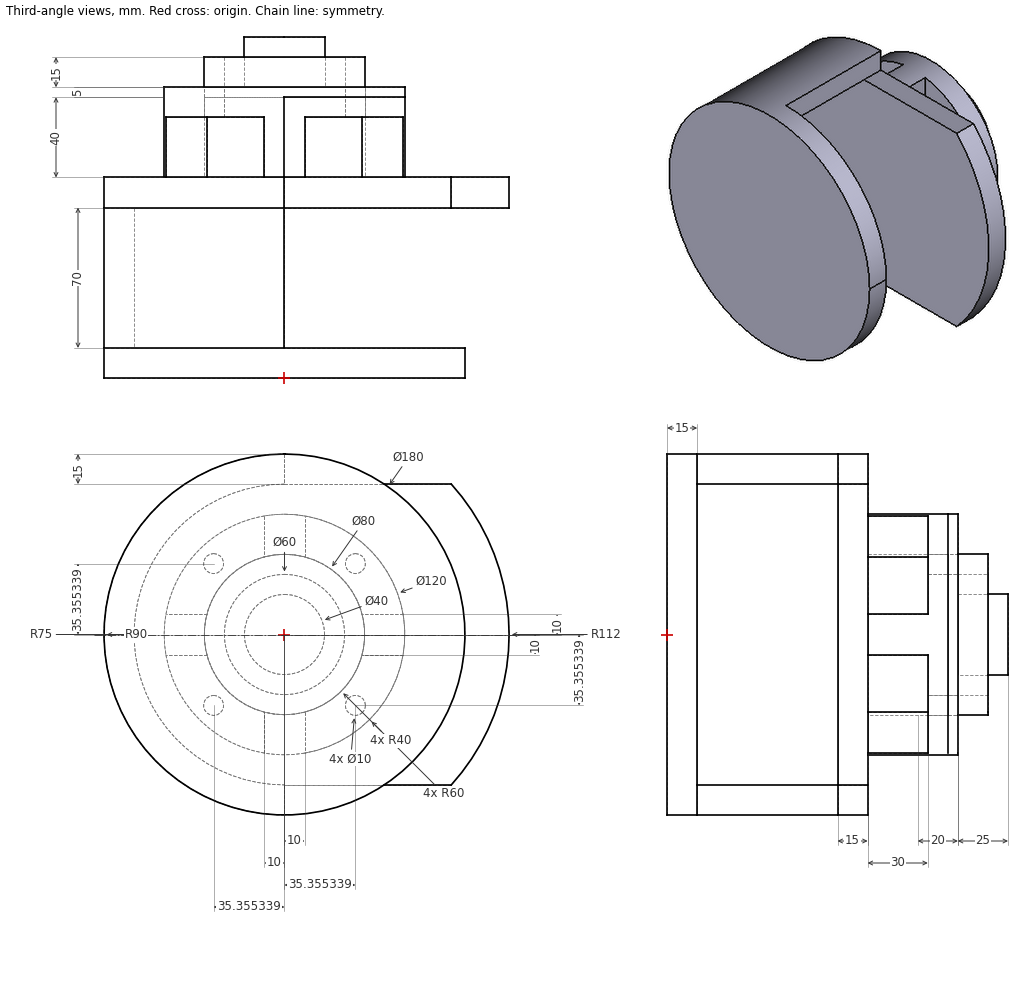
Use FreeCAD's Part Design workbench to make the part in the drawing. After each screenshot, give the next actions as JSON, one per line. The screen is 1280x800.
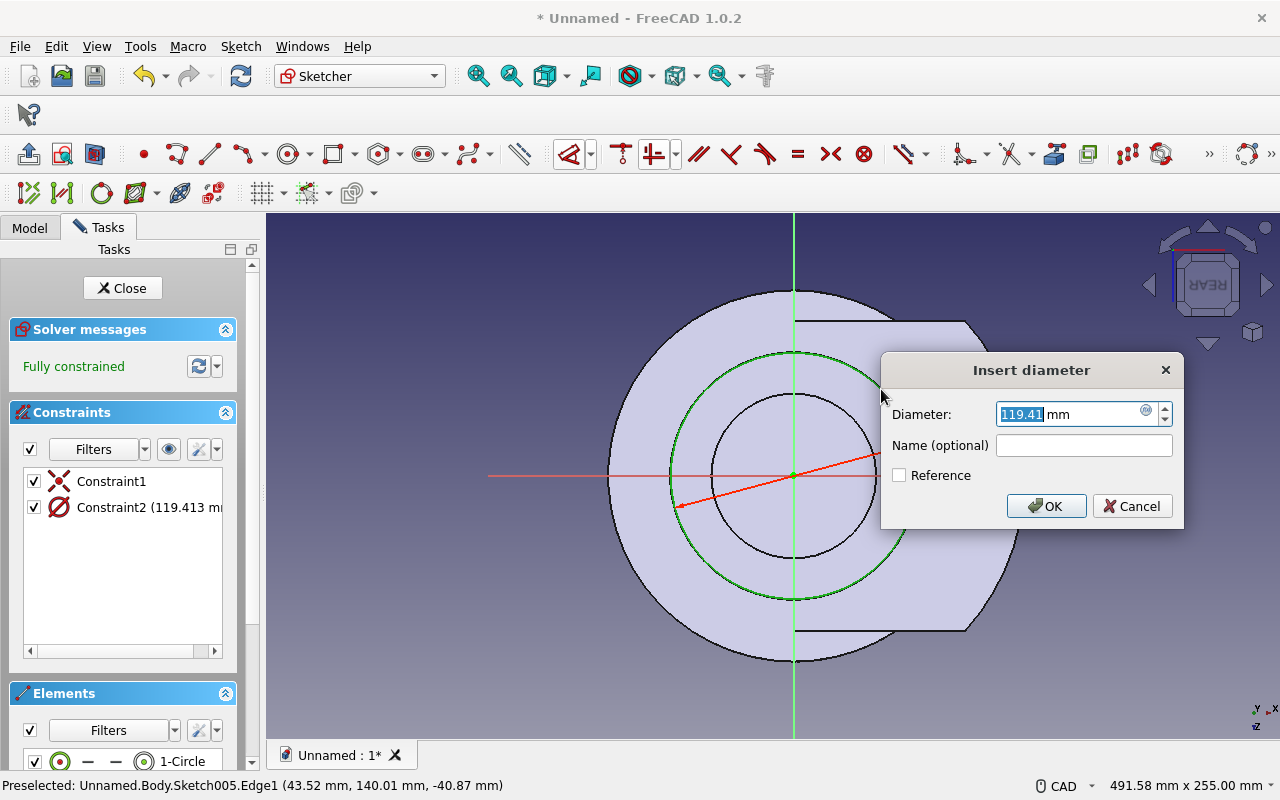
{"action": "type", "text": "120"}
{"action": "key", "text": "Return"}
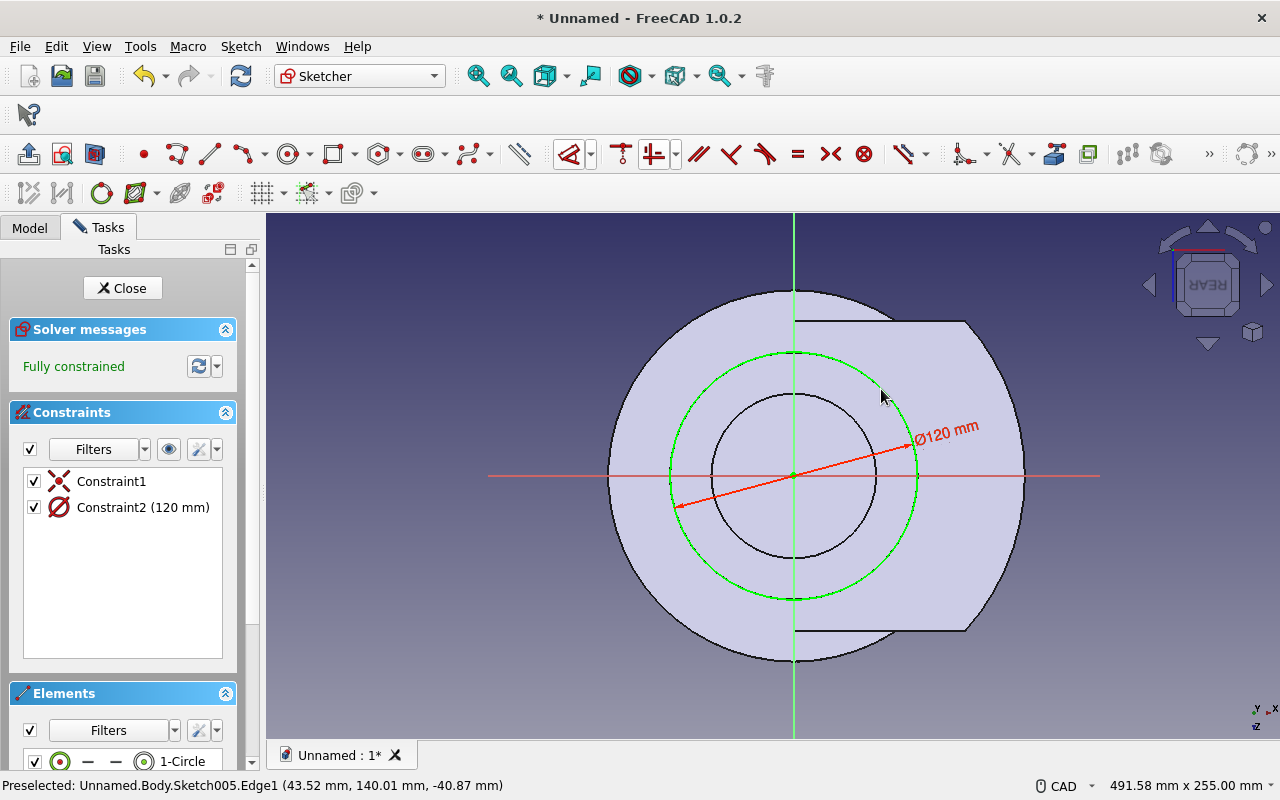
{"action": "left_click", "coordinate": [123, 288]}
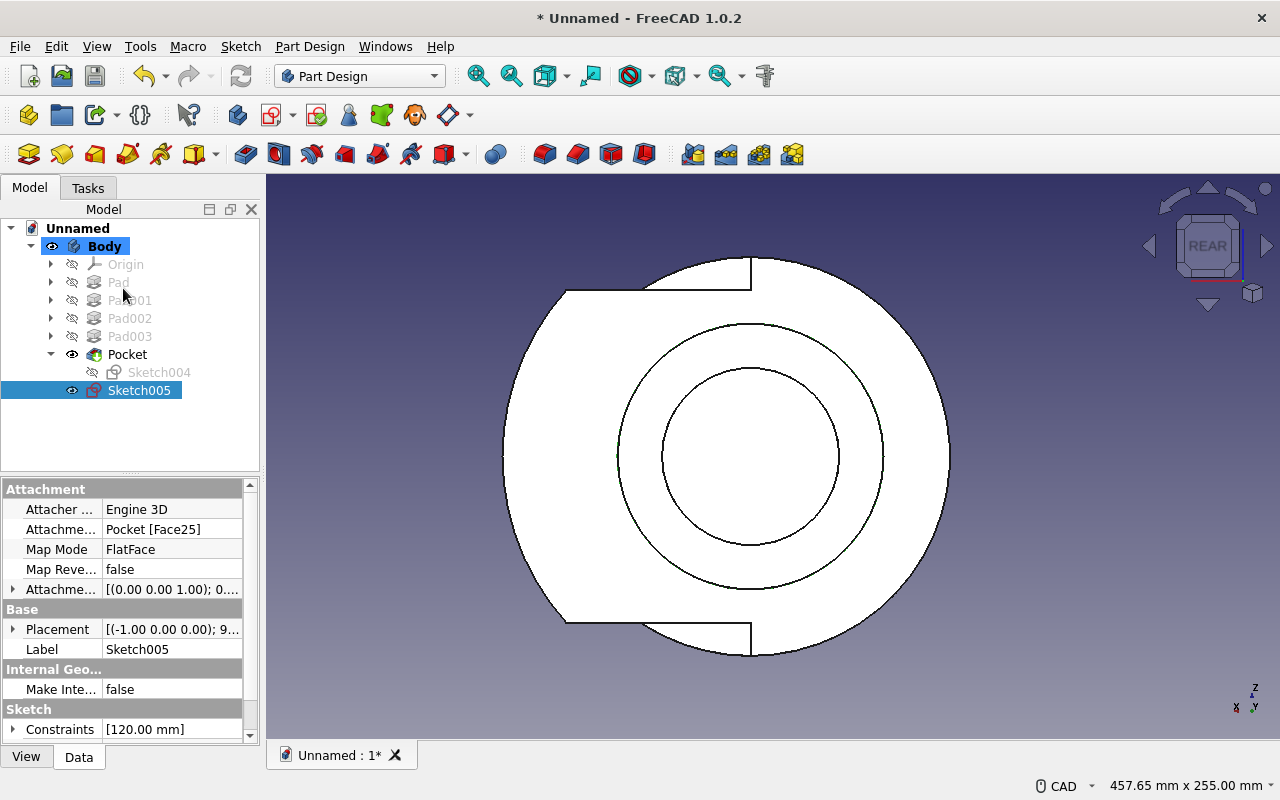
{"action": "left_click", "coordinate": [29, 154]}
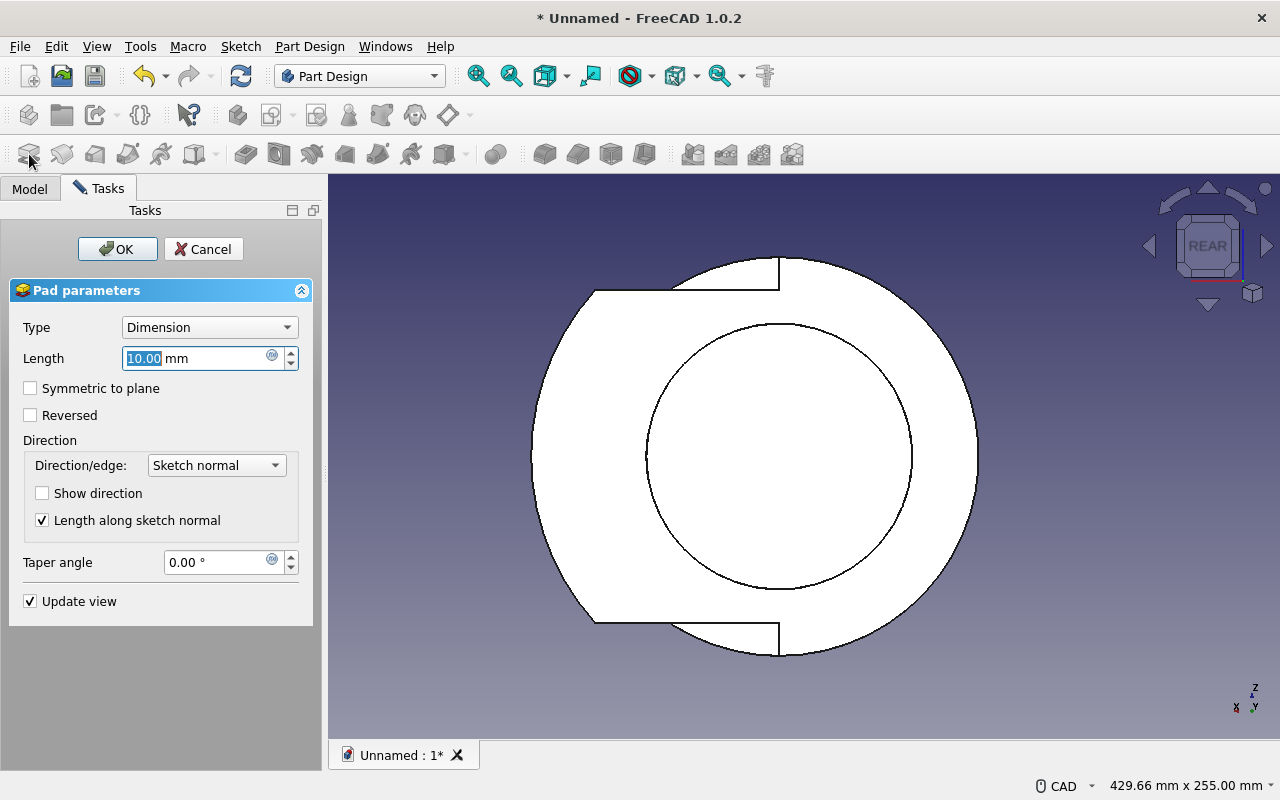
{"action": "type", "text": "5"}
{"action": "key", "text": "Tab"}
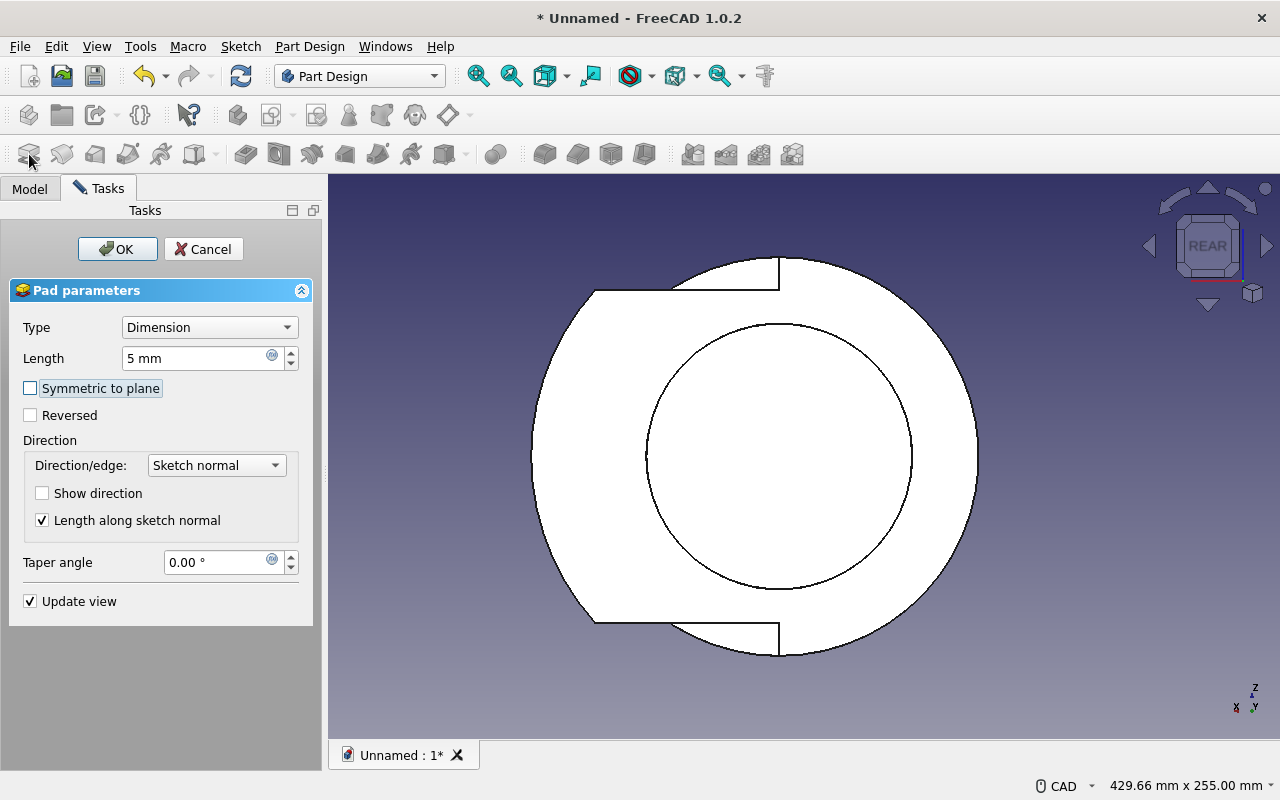
{"action": "left_click", "coordinate": [118, 249]}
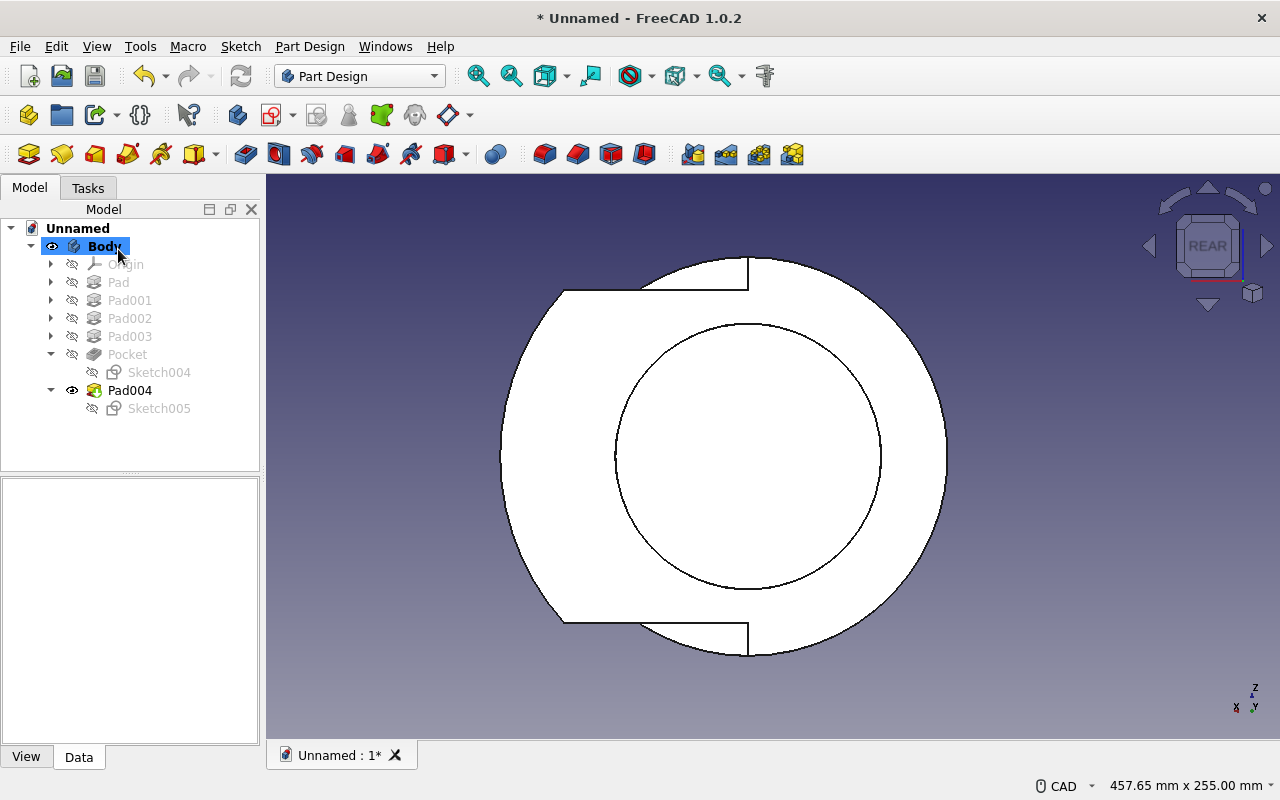
{"action": "left_click", "coordinate": [748, 455]}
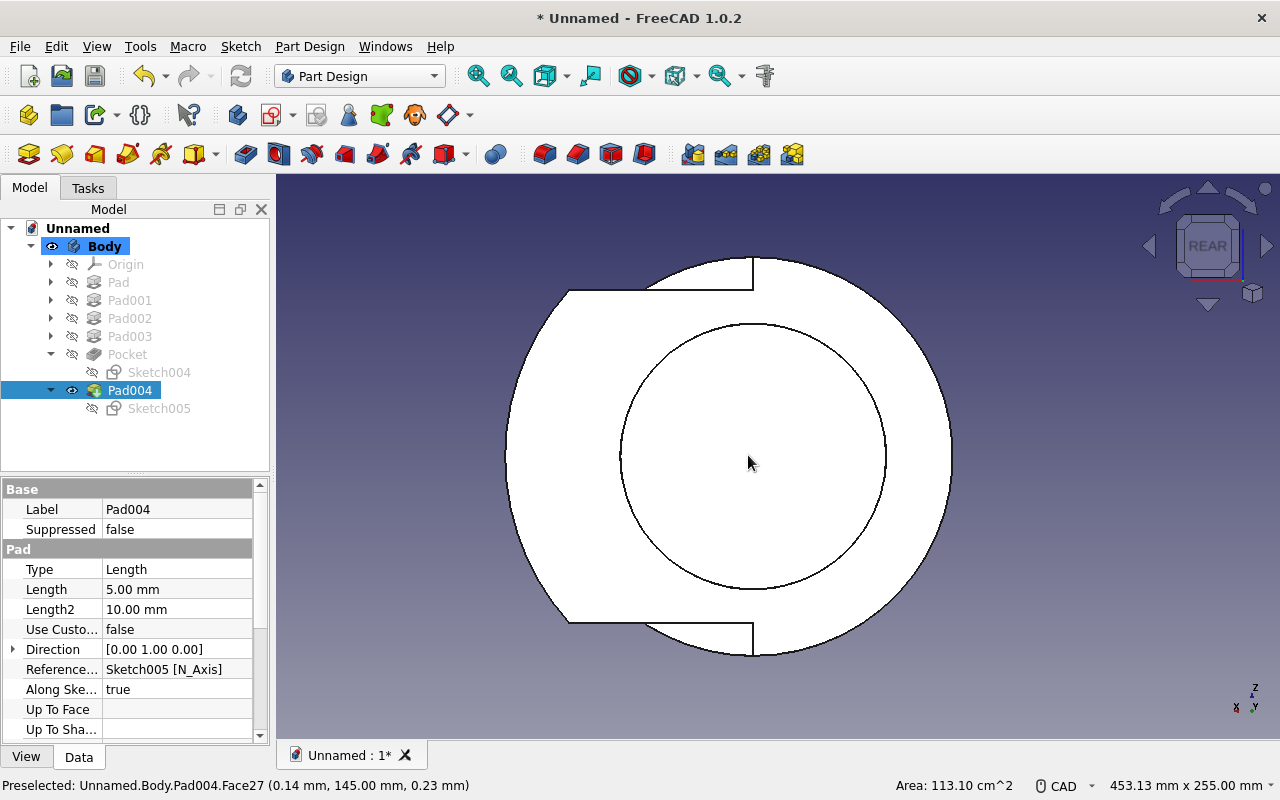
{"action": "left_click", "coordinate": [270, 116]}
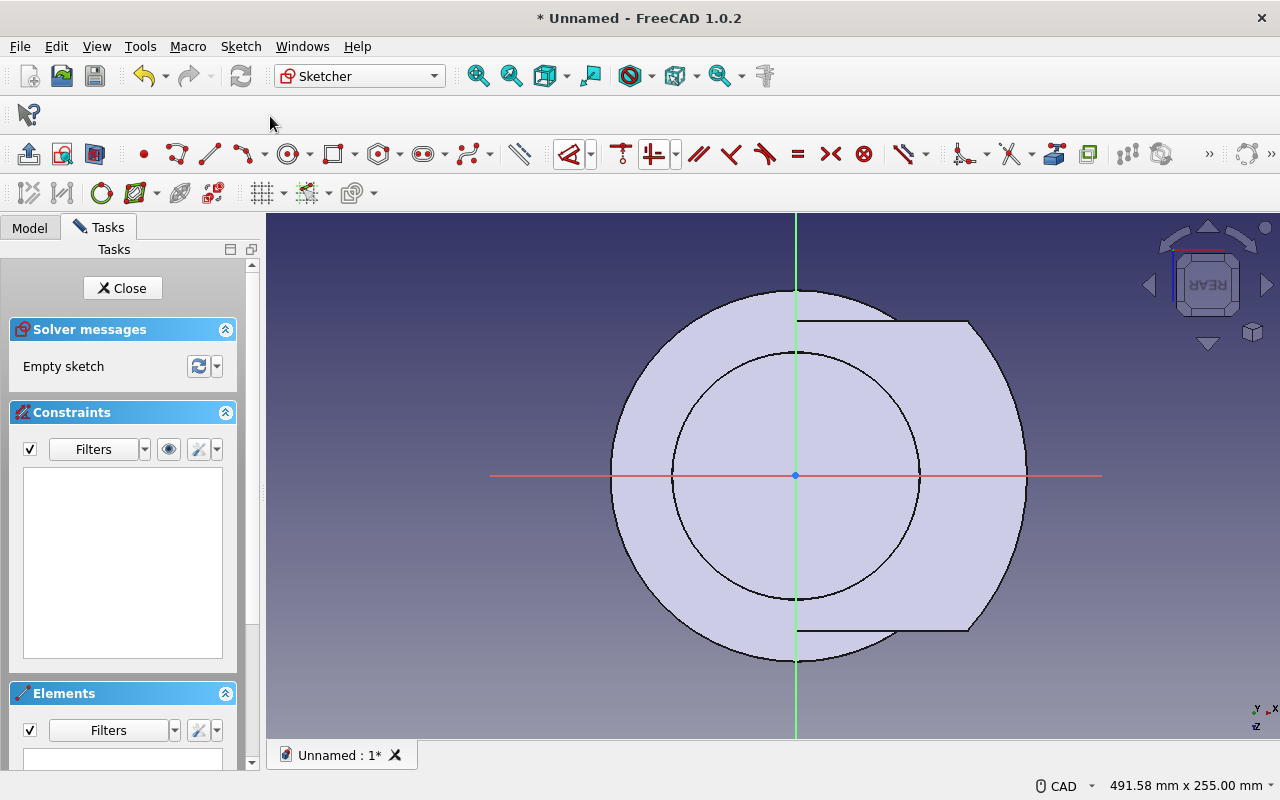
{"action": "scroll", "coordinate": [907, 476], "scroll_direction": "up", "scroll_amount": 3}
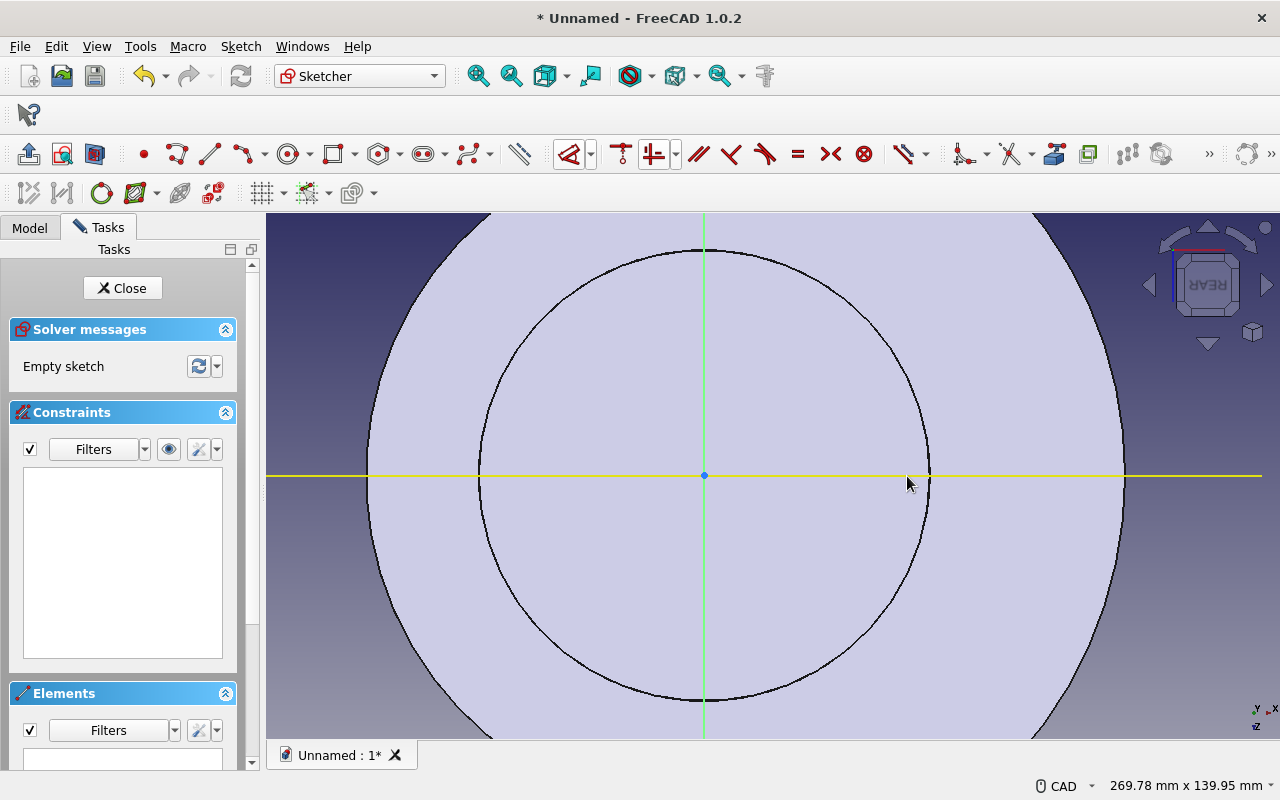
{"action": "left_click", "coordinate": [288, 154]}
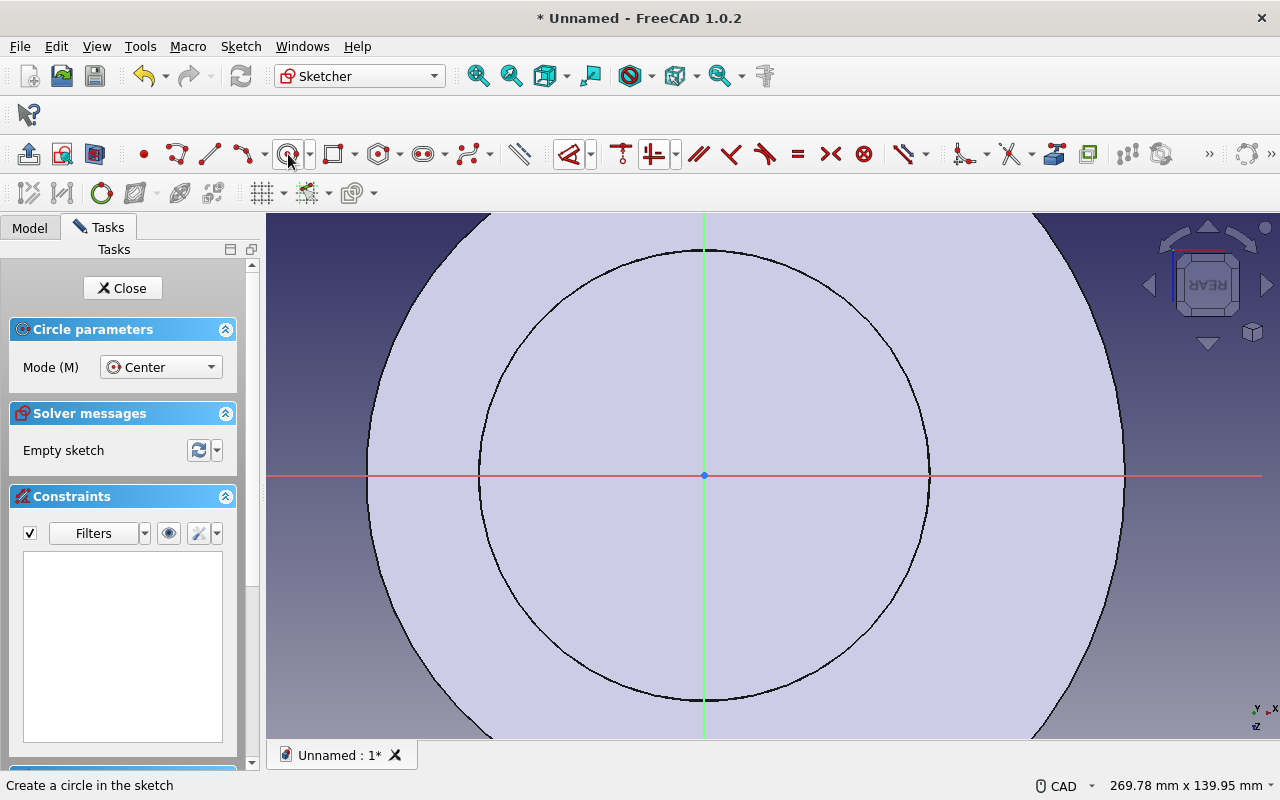
{"action": "left_click", "coordinate": [837, 343]}
{"action": "left_click", "coordinate": [850, 329]}